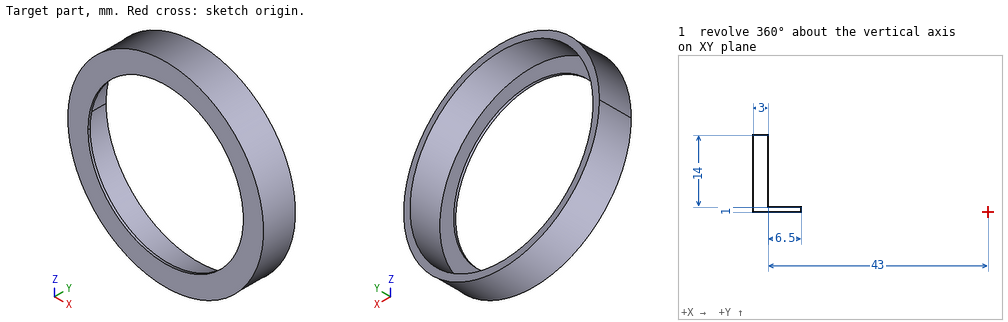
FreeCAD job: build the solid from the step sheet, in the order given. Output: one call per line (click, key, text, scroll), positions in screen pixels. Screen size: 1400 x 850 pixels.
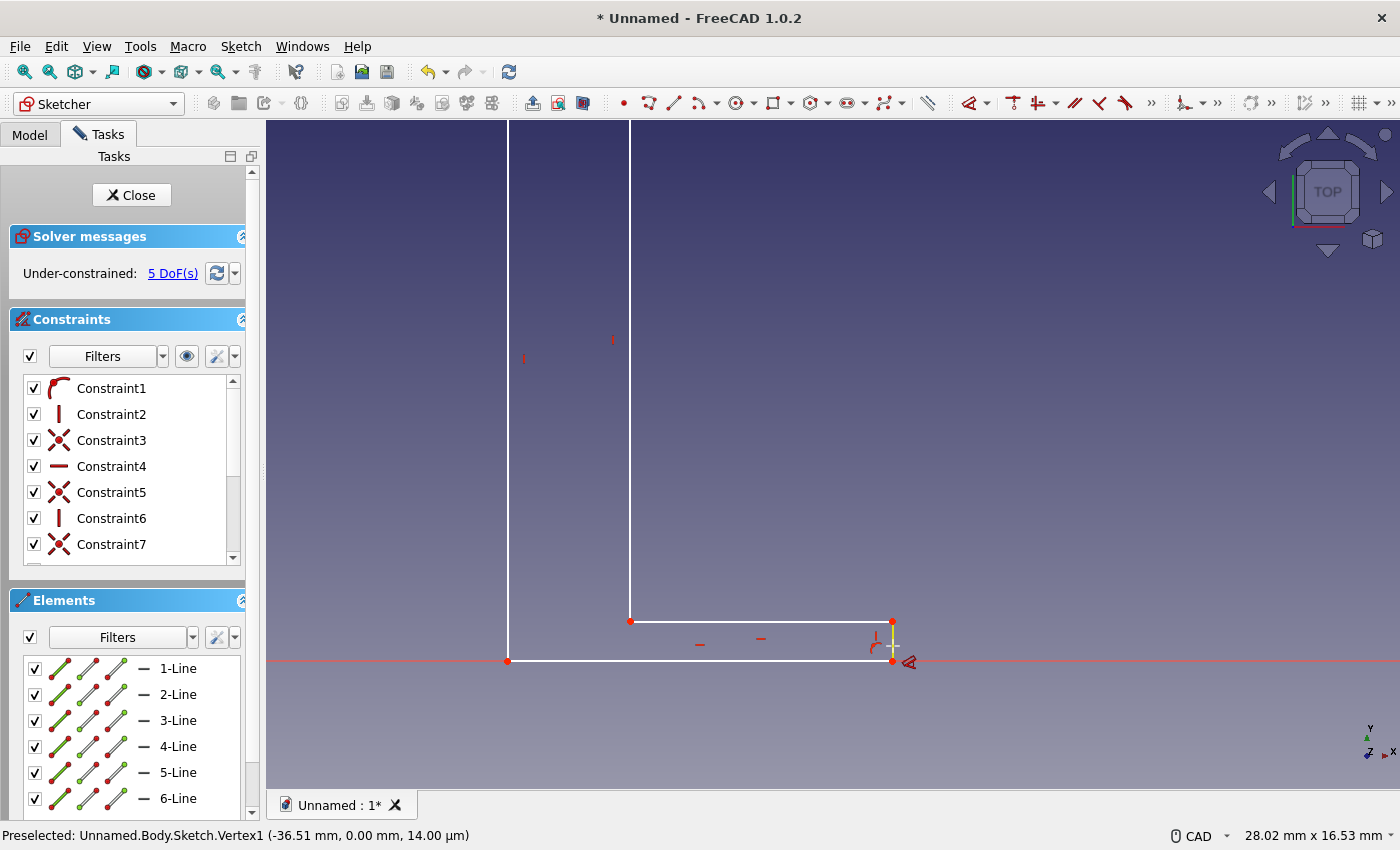
click(893, 645)
click(927, 641)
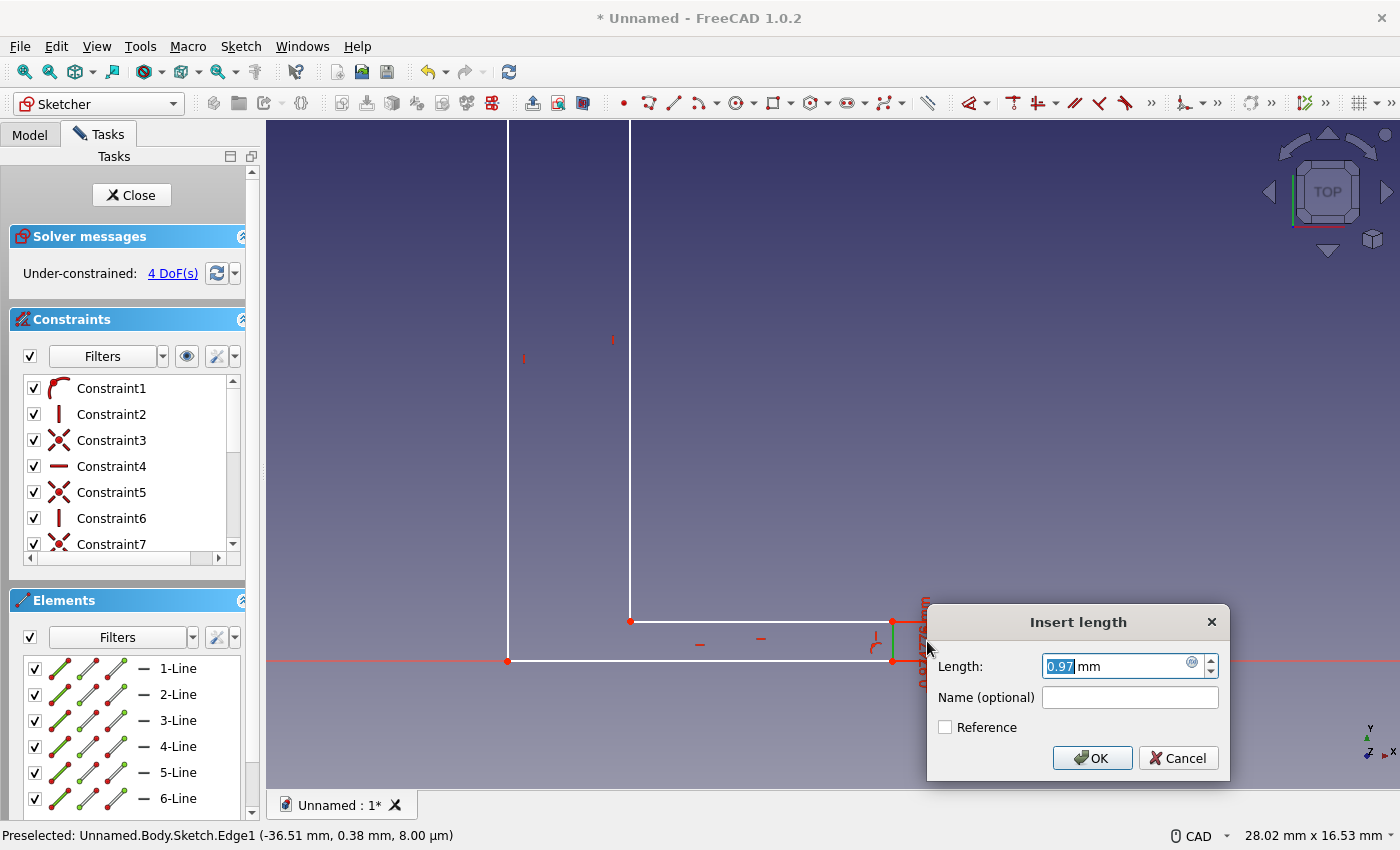
text(1)
key(Return)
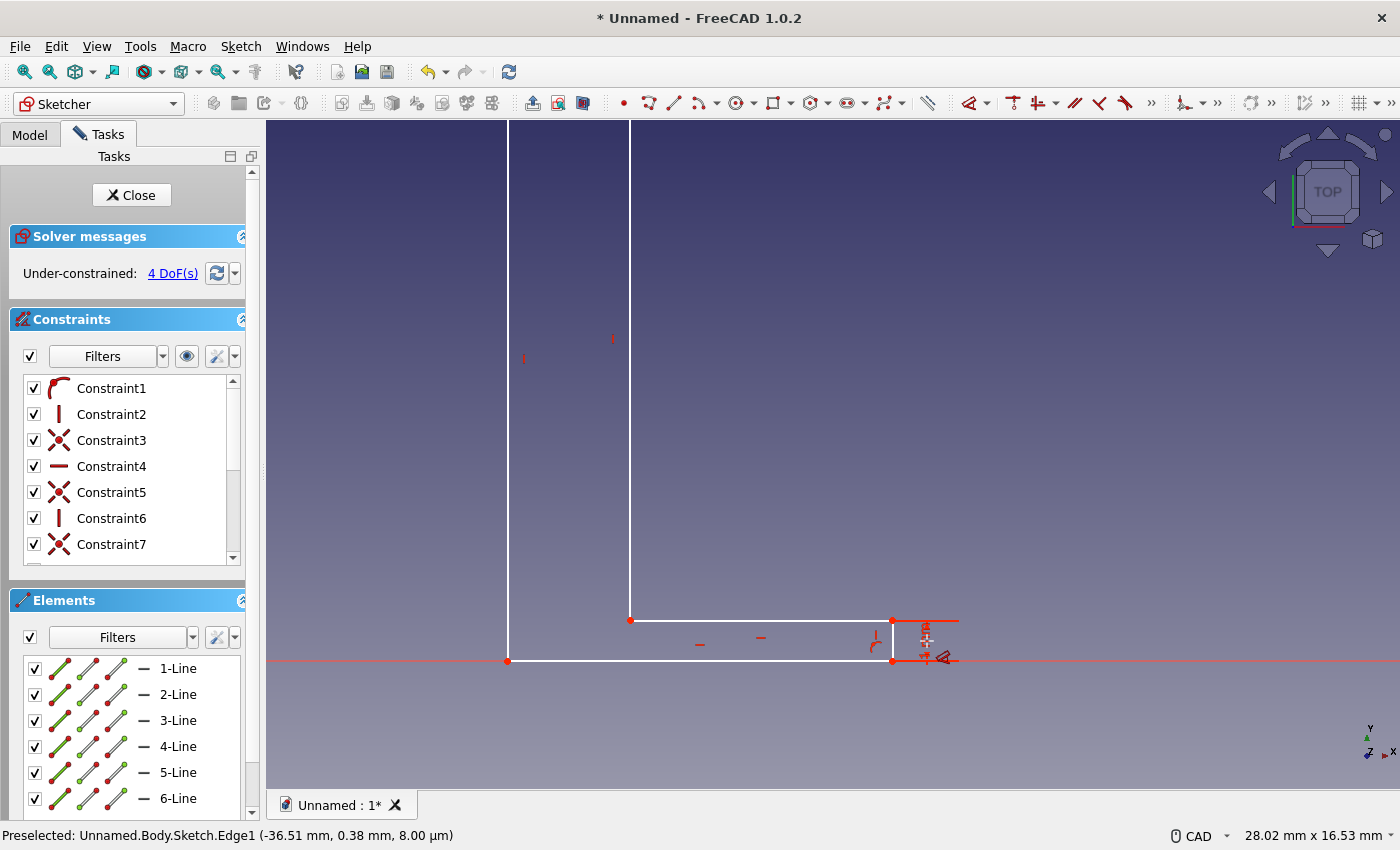
scroll(894, 651, down, 2)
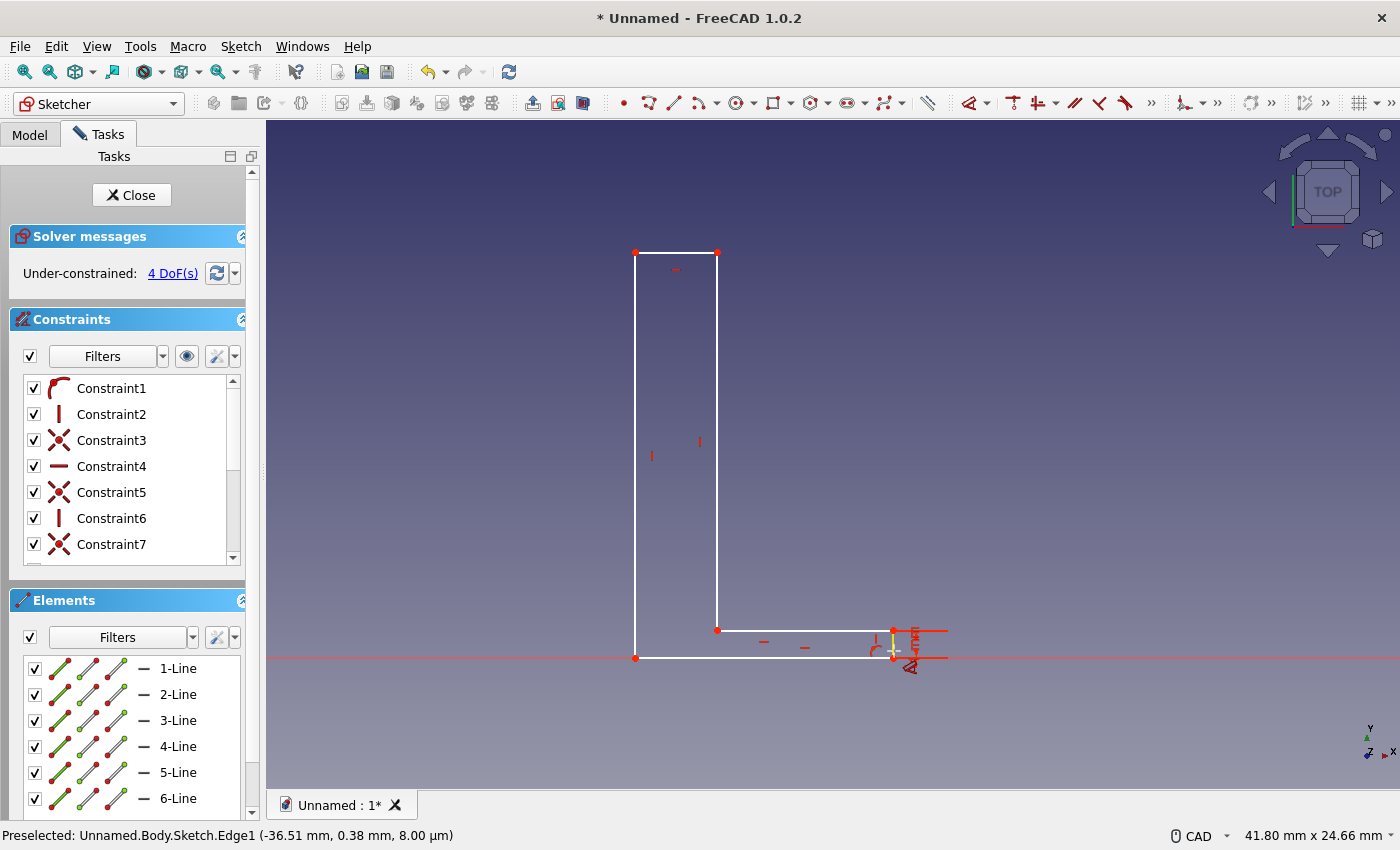
click(693, 253)
click(676, 219)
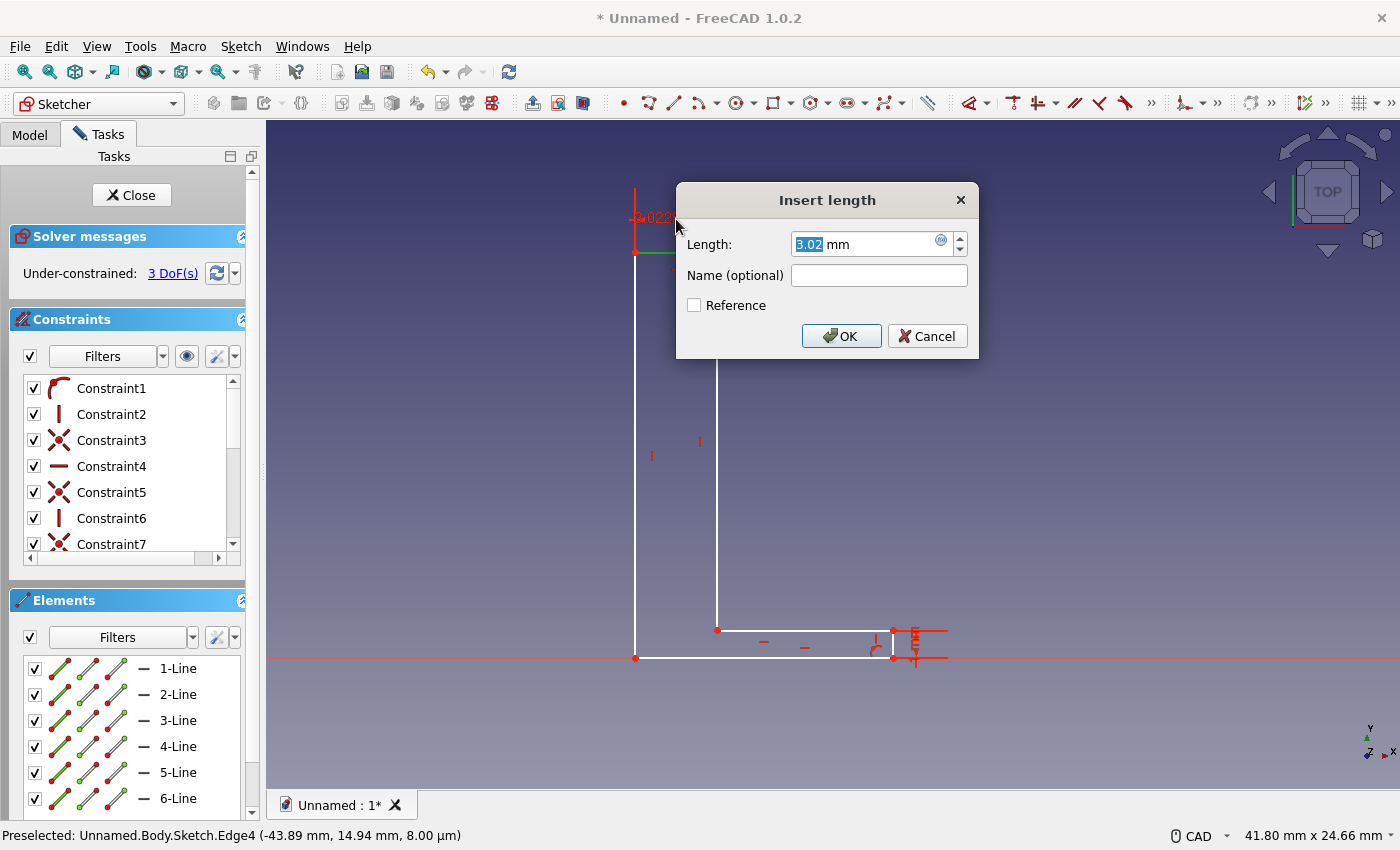
text(3)
key(Return)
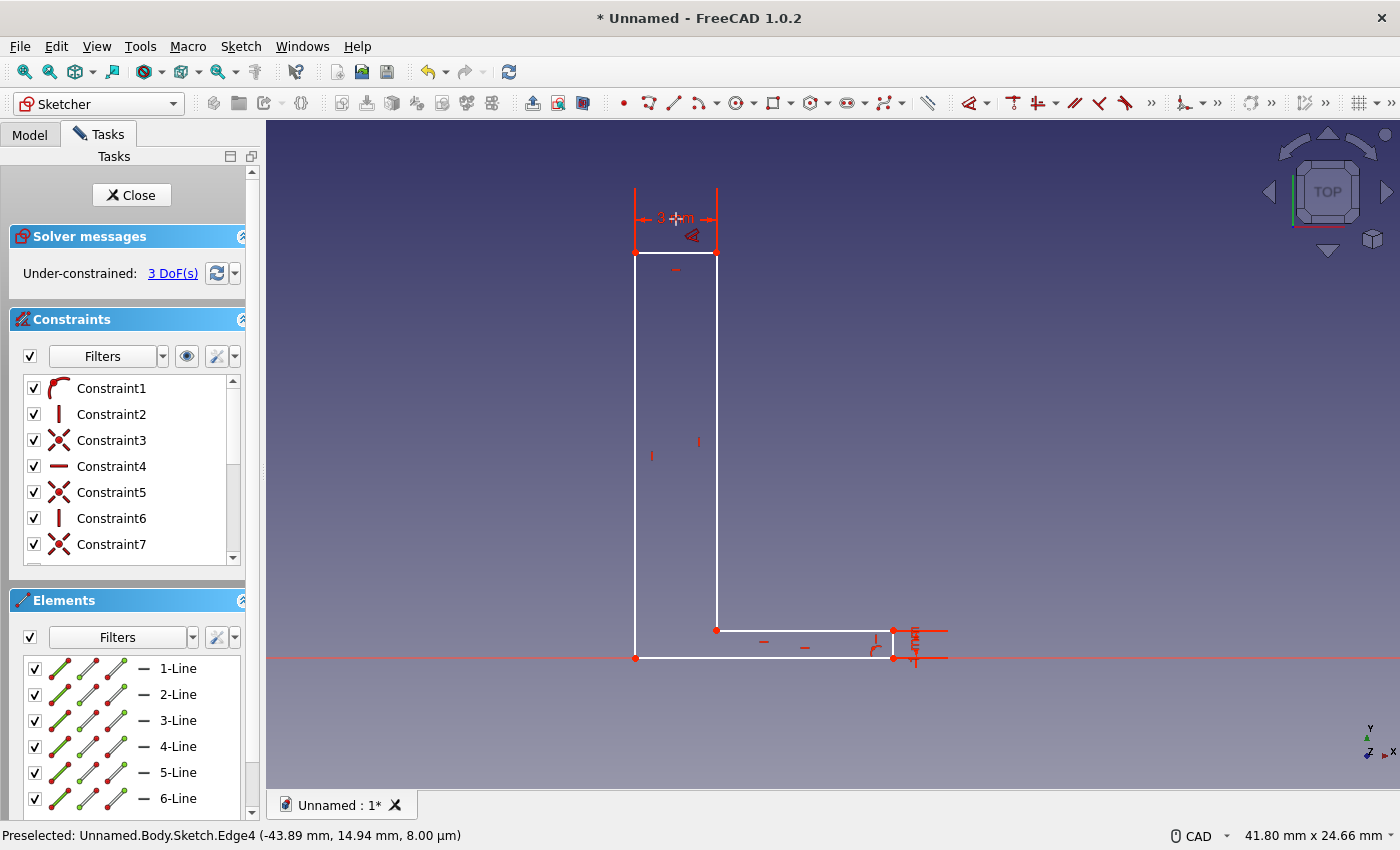
click(717, 517)
click(683, 442)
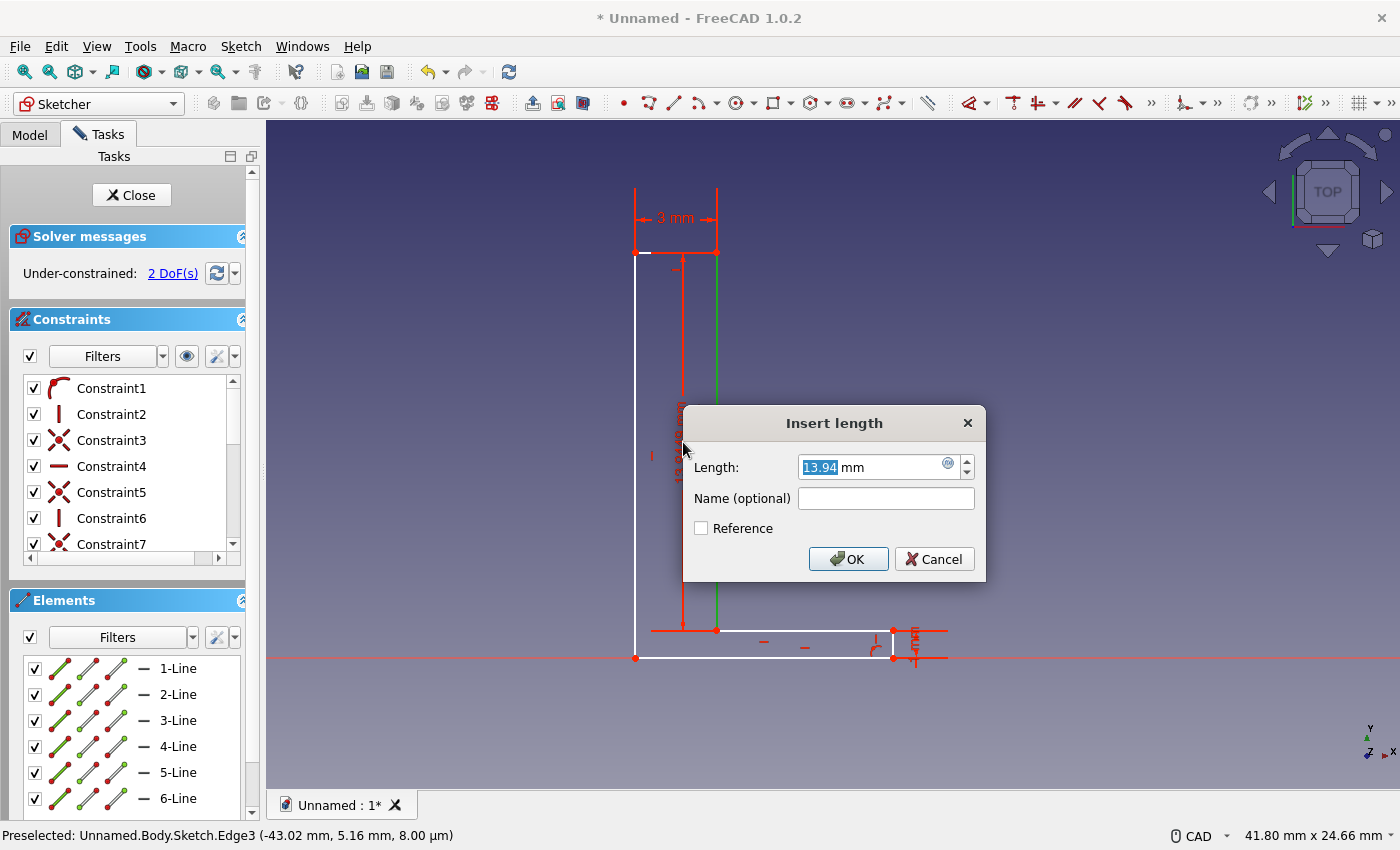
text(14)
key(Return)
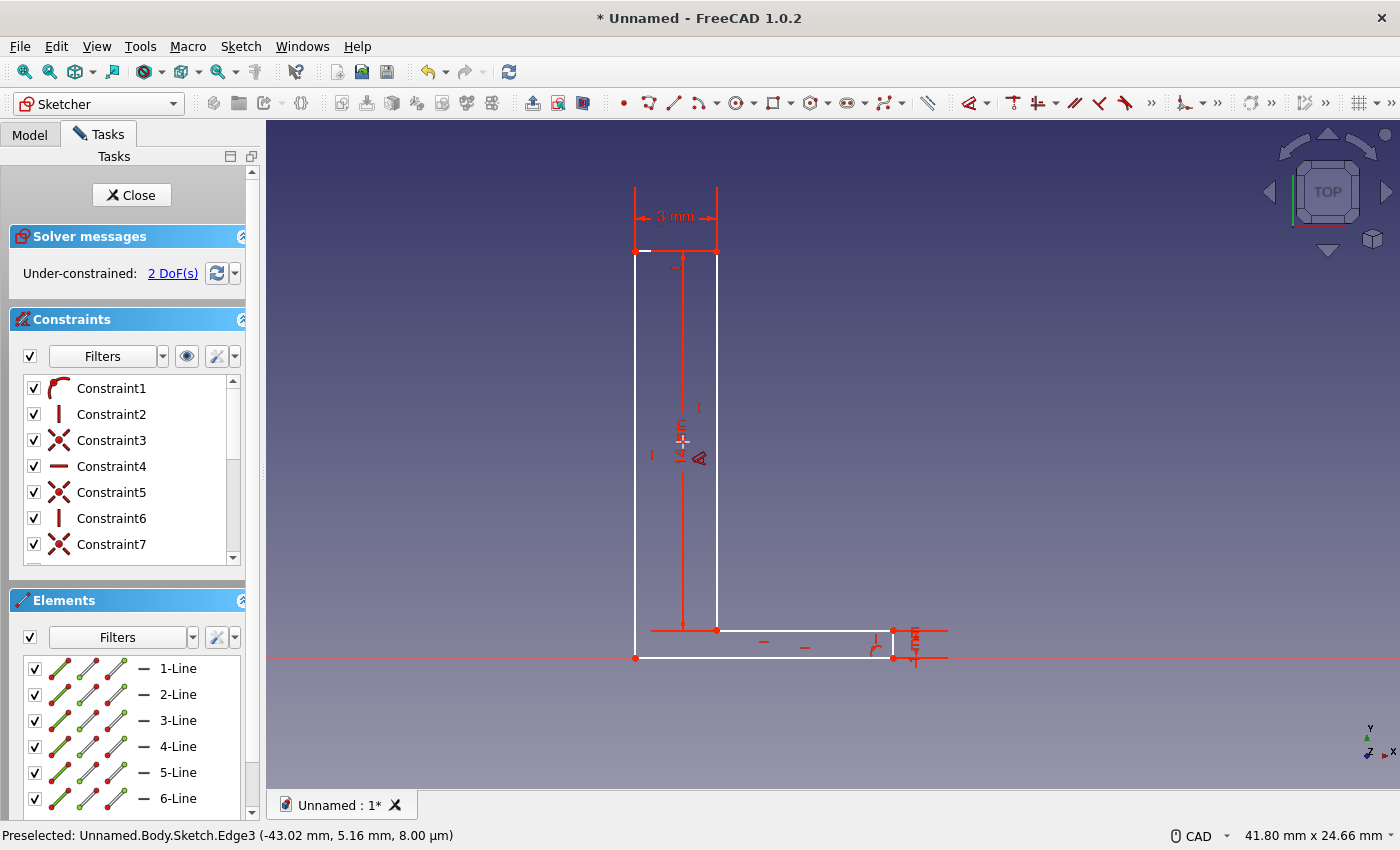
click(840, 631)
click(805, 597)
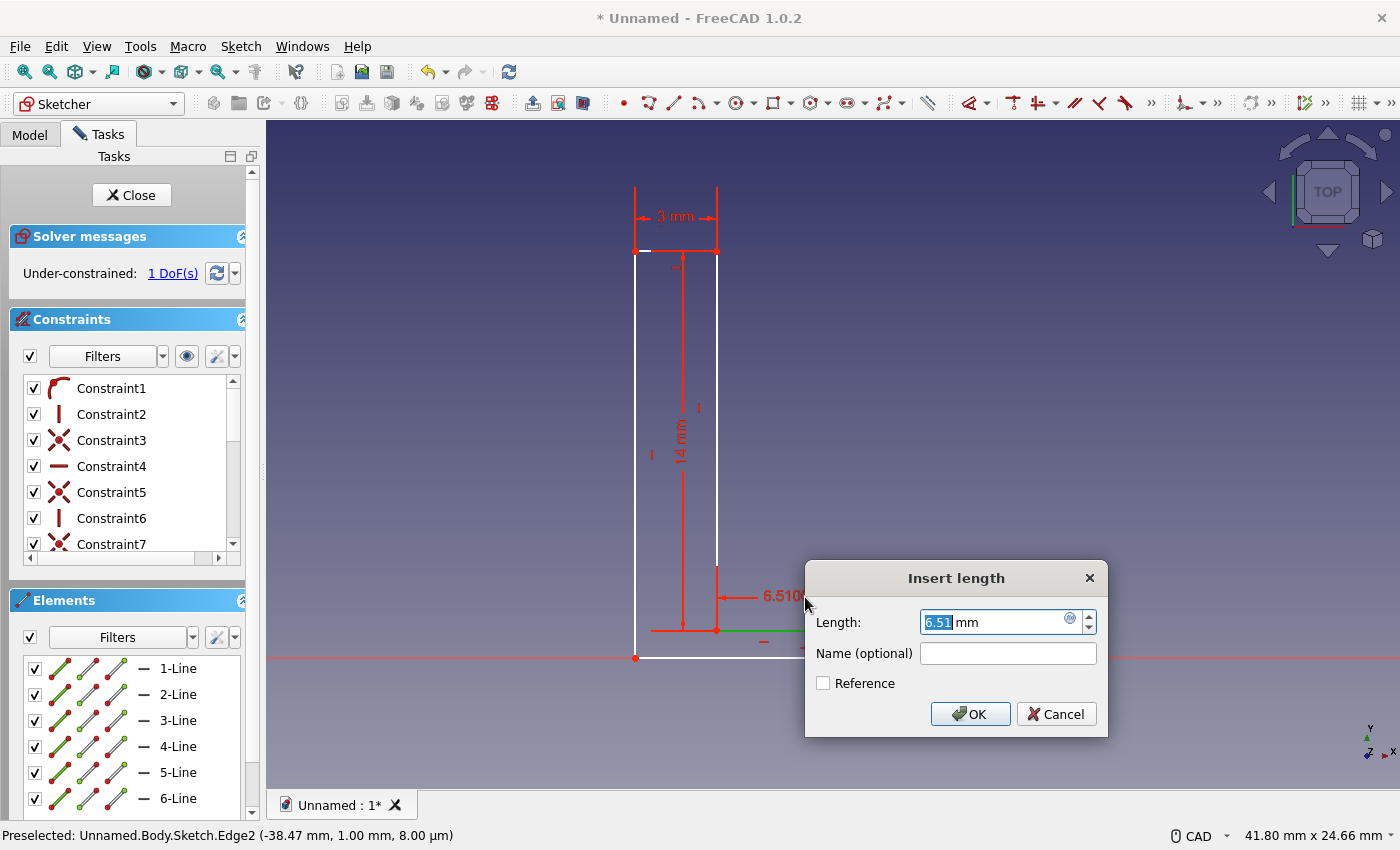
text(6.5)
key(Return)